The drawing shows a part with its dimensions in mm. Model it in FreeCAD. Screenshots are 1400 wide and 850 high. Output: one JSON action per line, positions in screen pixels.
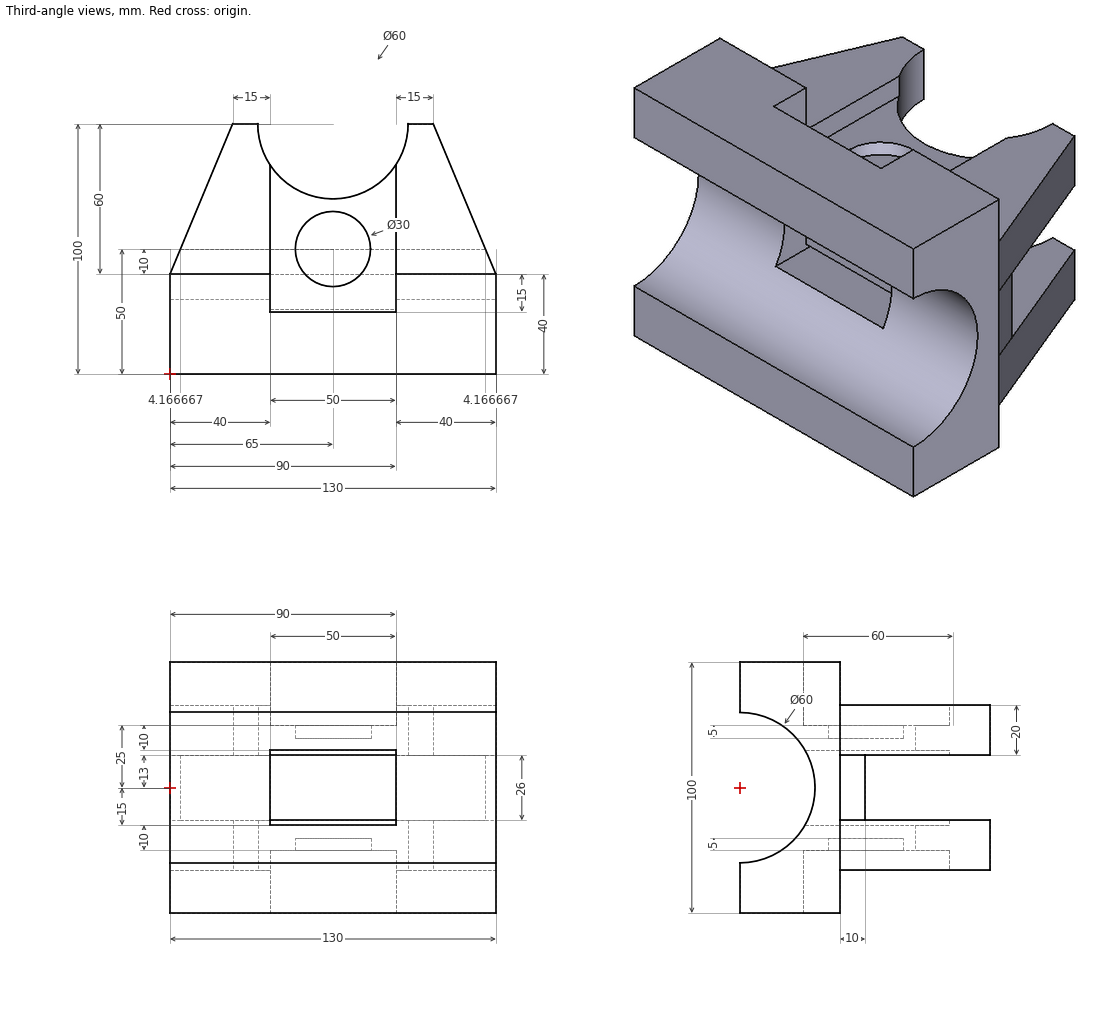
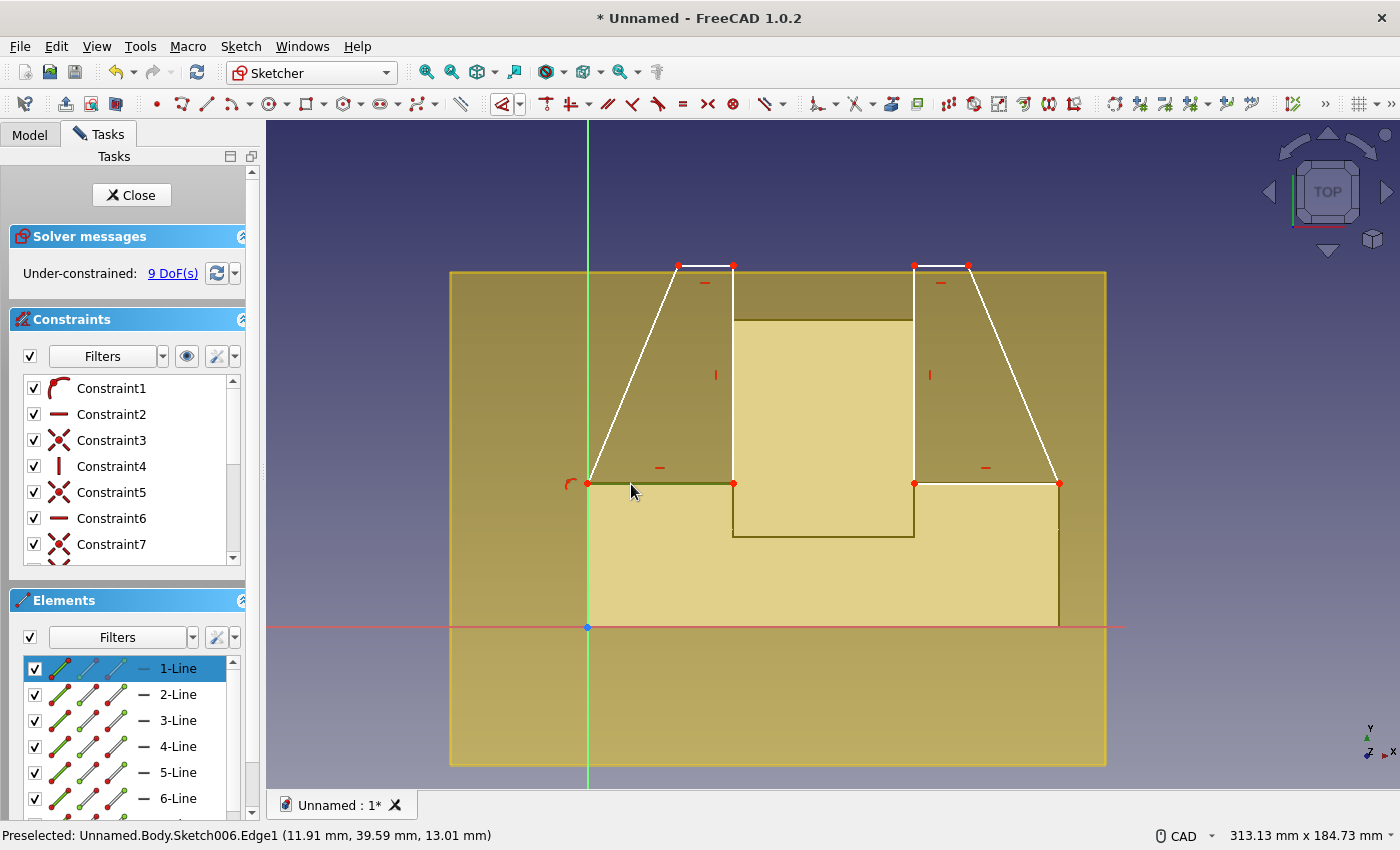
{"action": "left_click", "coordinate": [520, 104]}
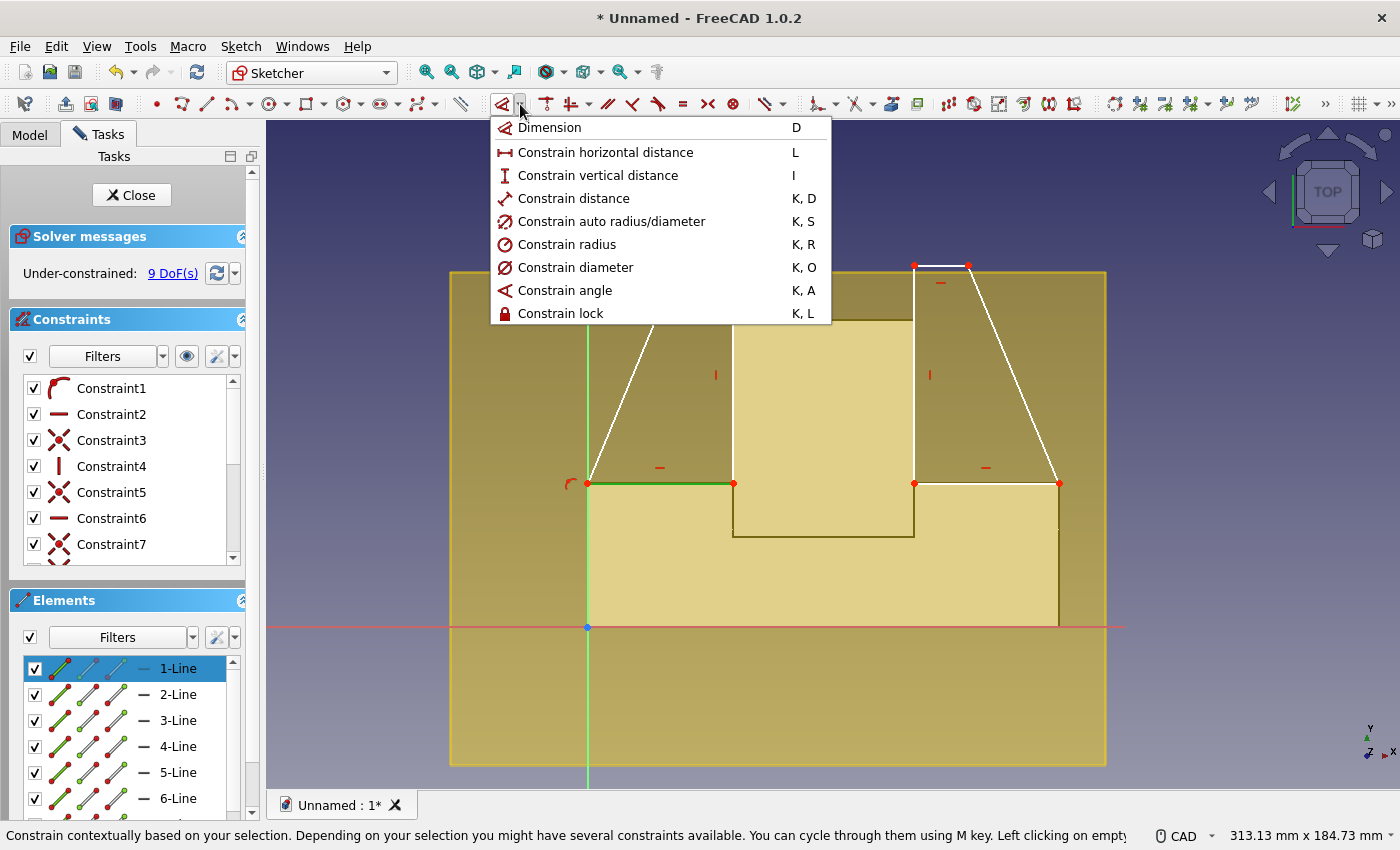
{"action": "left_click", "coordinate": [661, 152]}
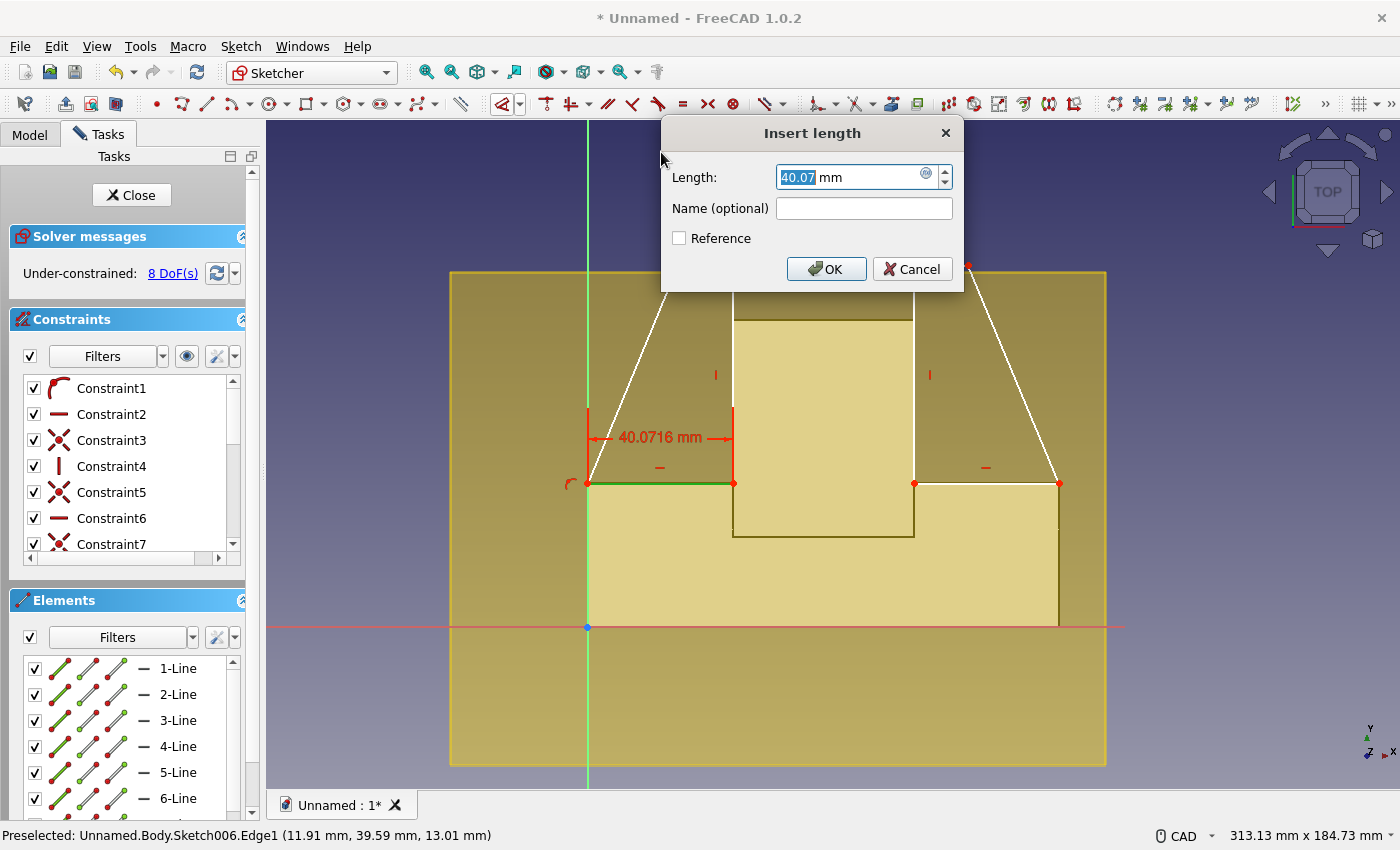
{"action": "type", "text": "40"}
{"action": "key", "text": "Return"}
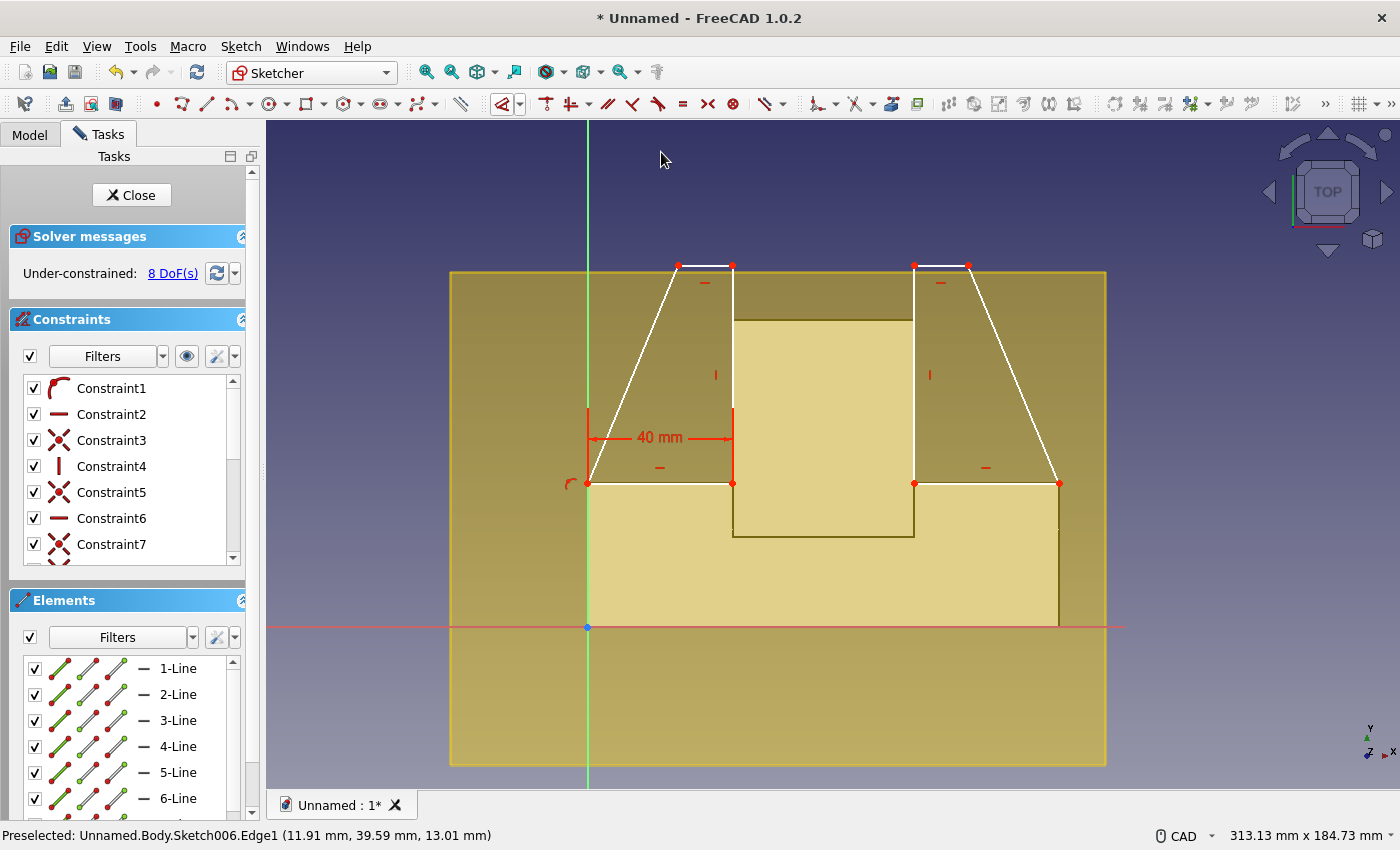
{"action": "left_click", "coordinate": [733, 419]}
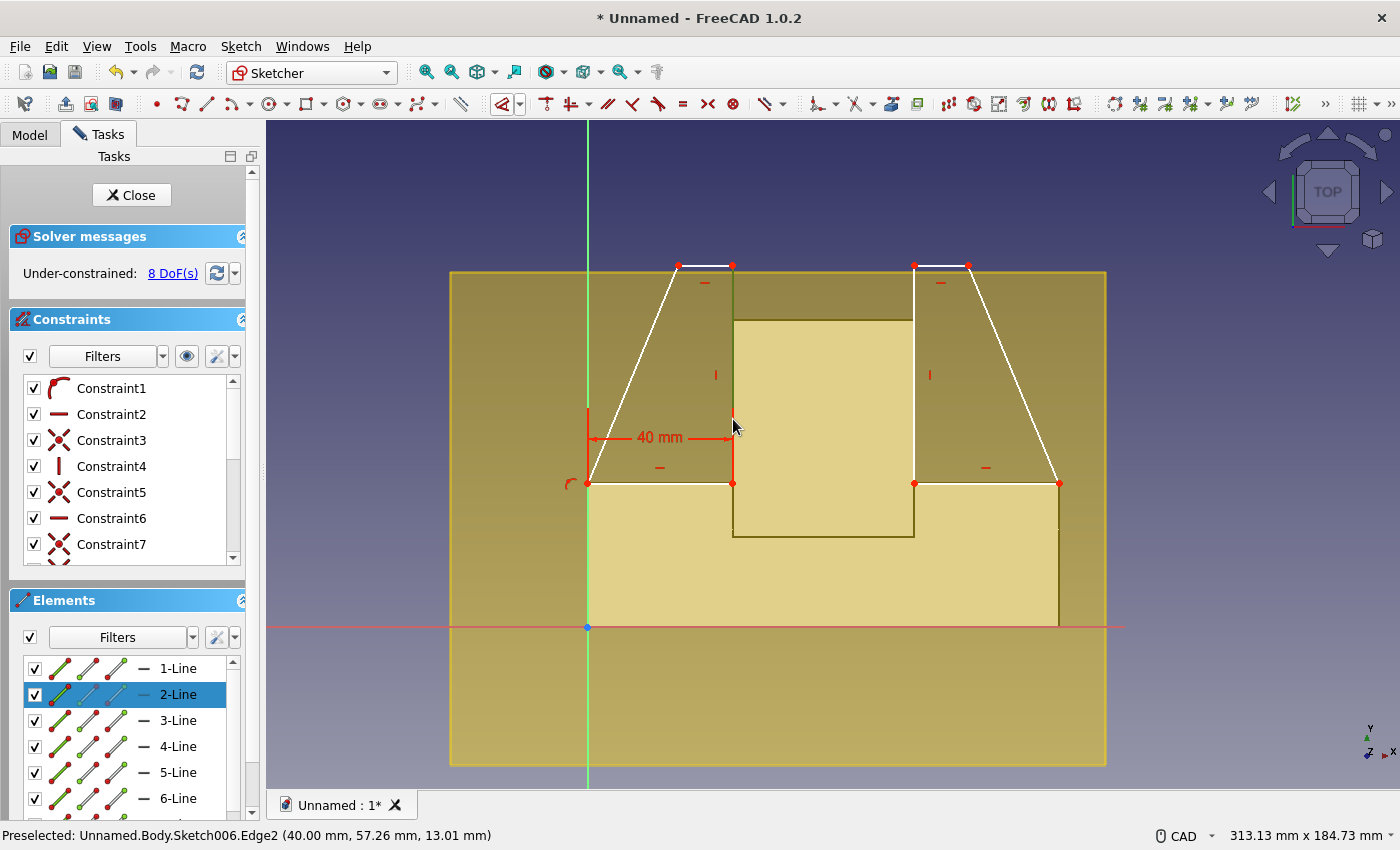
{"action": "key", "text": "i"}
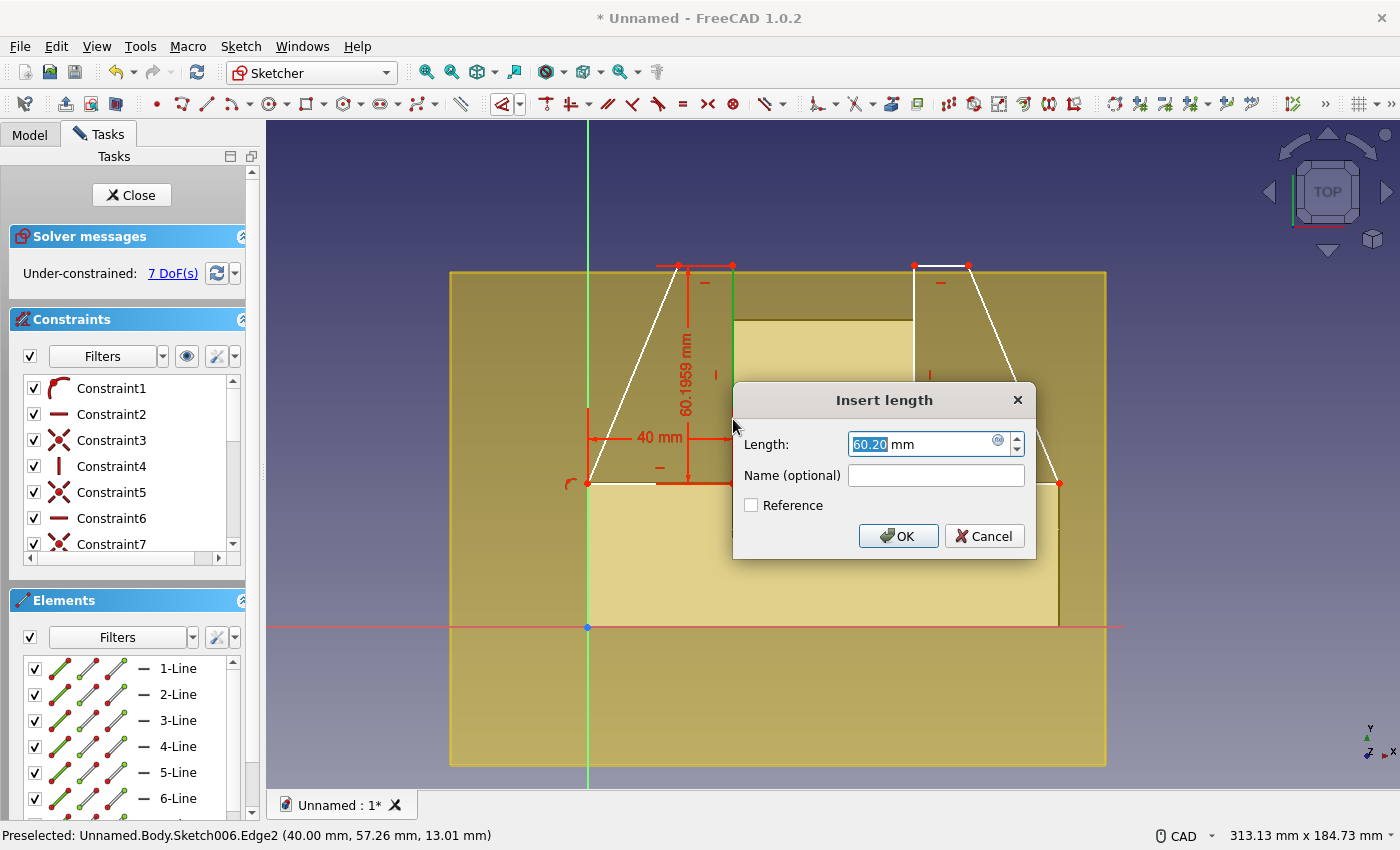
{"action": "type", "text": "60"}
{"action": "key", "text": "Return"}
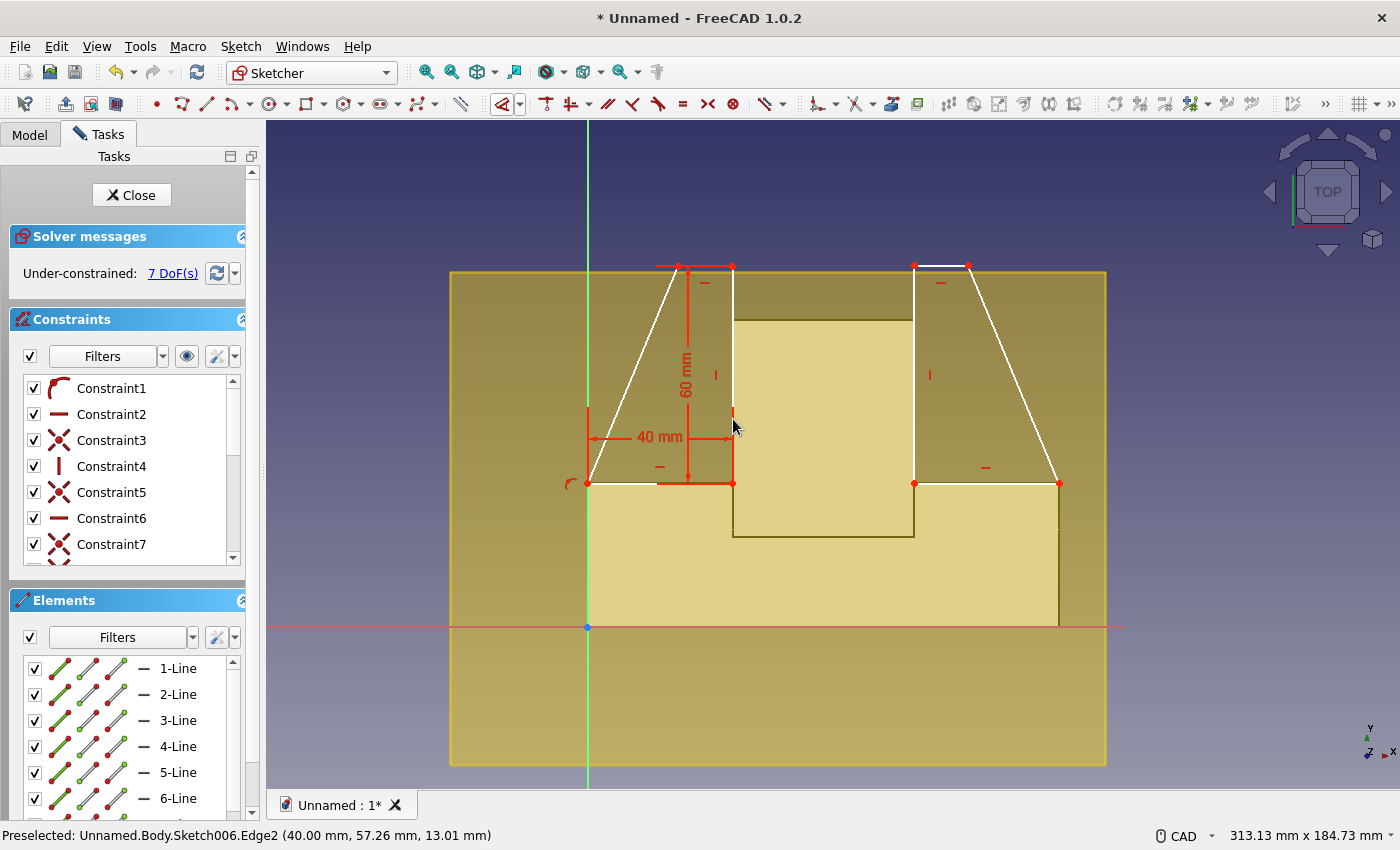
{"action": "left_click", "coordinate": [716, 266]}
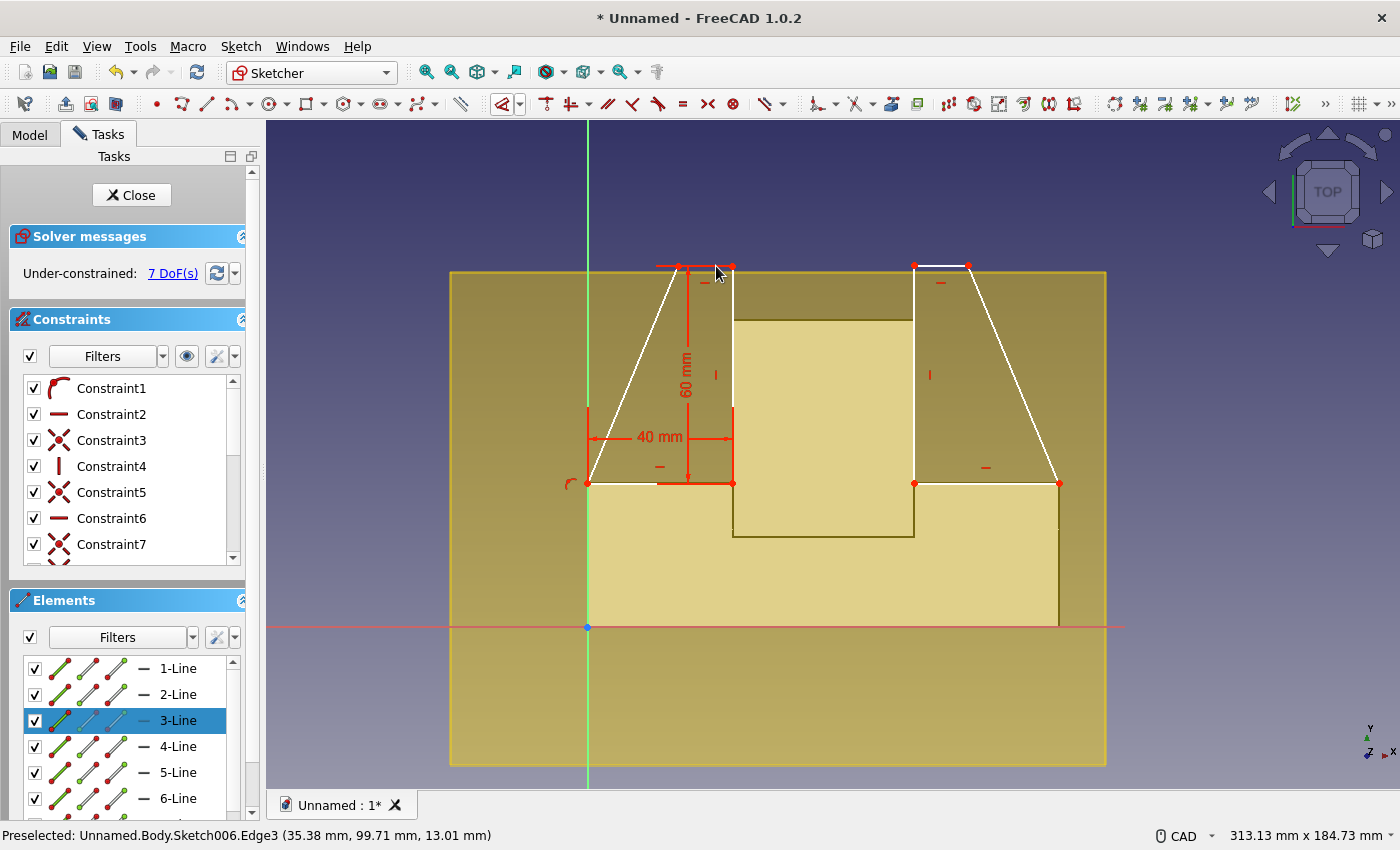
{"action": "left_click", "coordinate": [520, 104]}